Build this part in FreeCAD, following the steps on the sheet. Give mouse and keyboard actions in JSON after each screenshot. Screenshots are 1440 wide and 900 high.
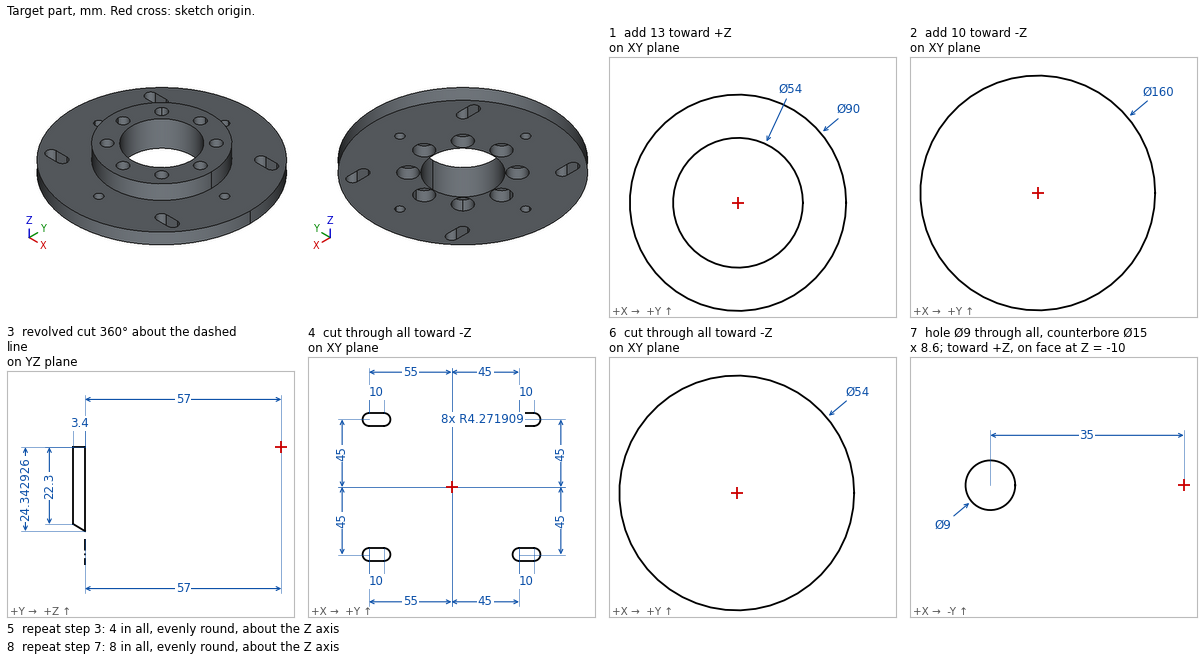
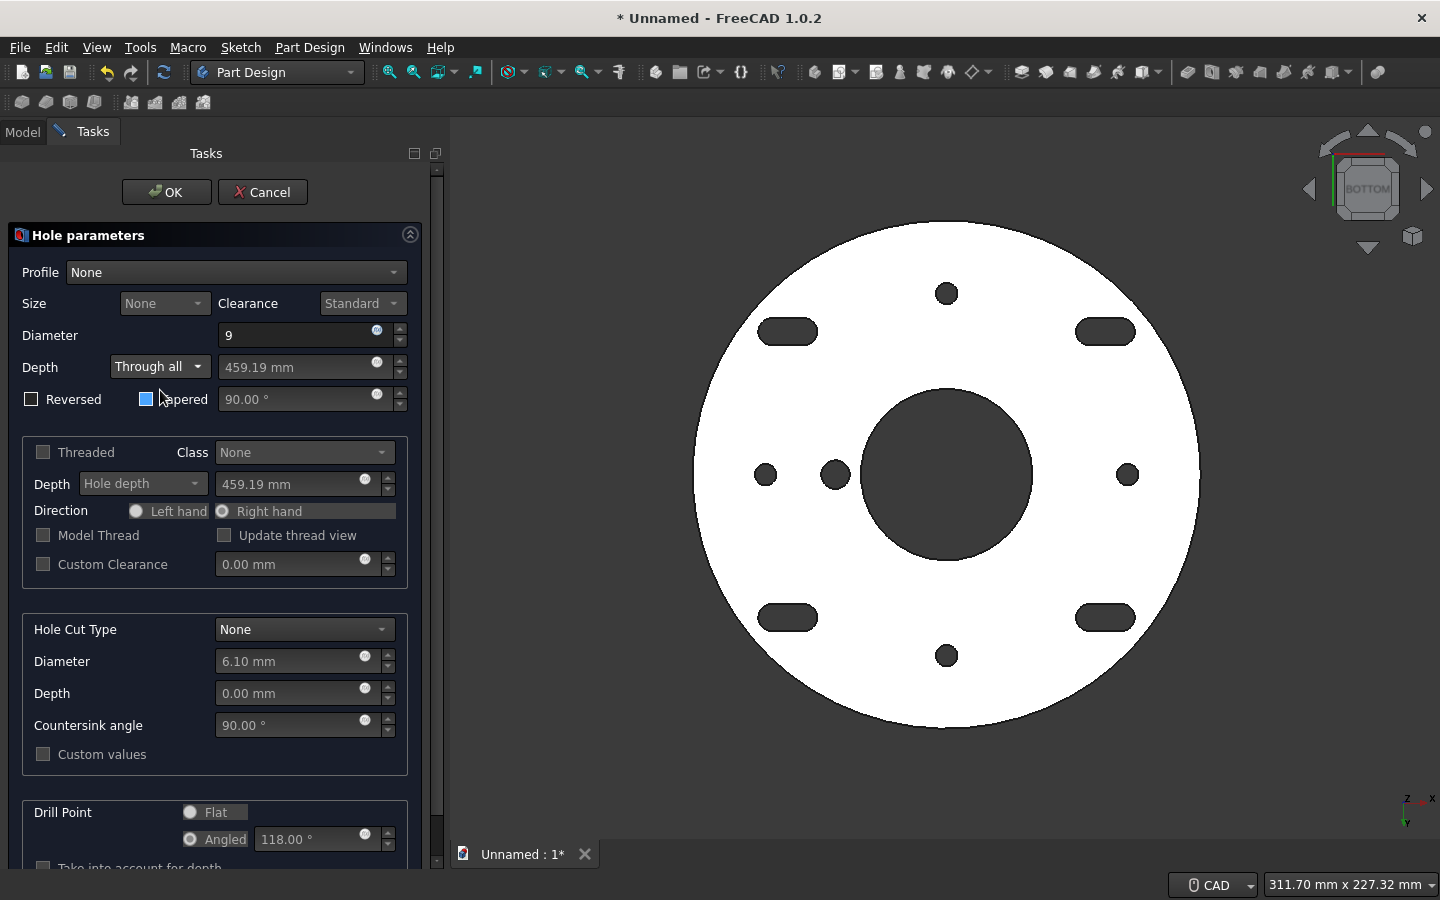
{"action": "left_click", "coordinate": [306, 630]}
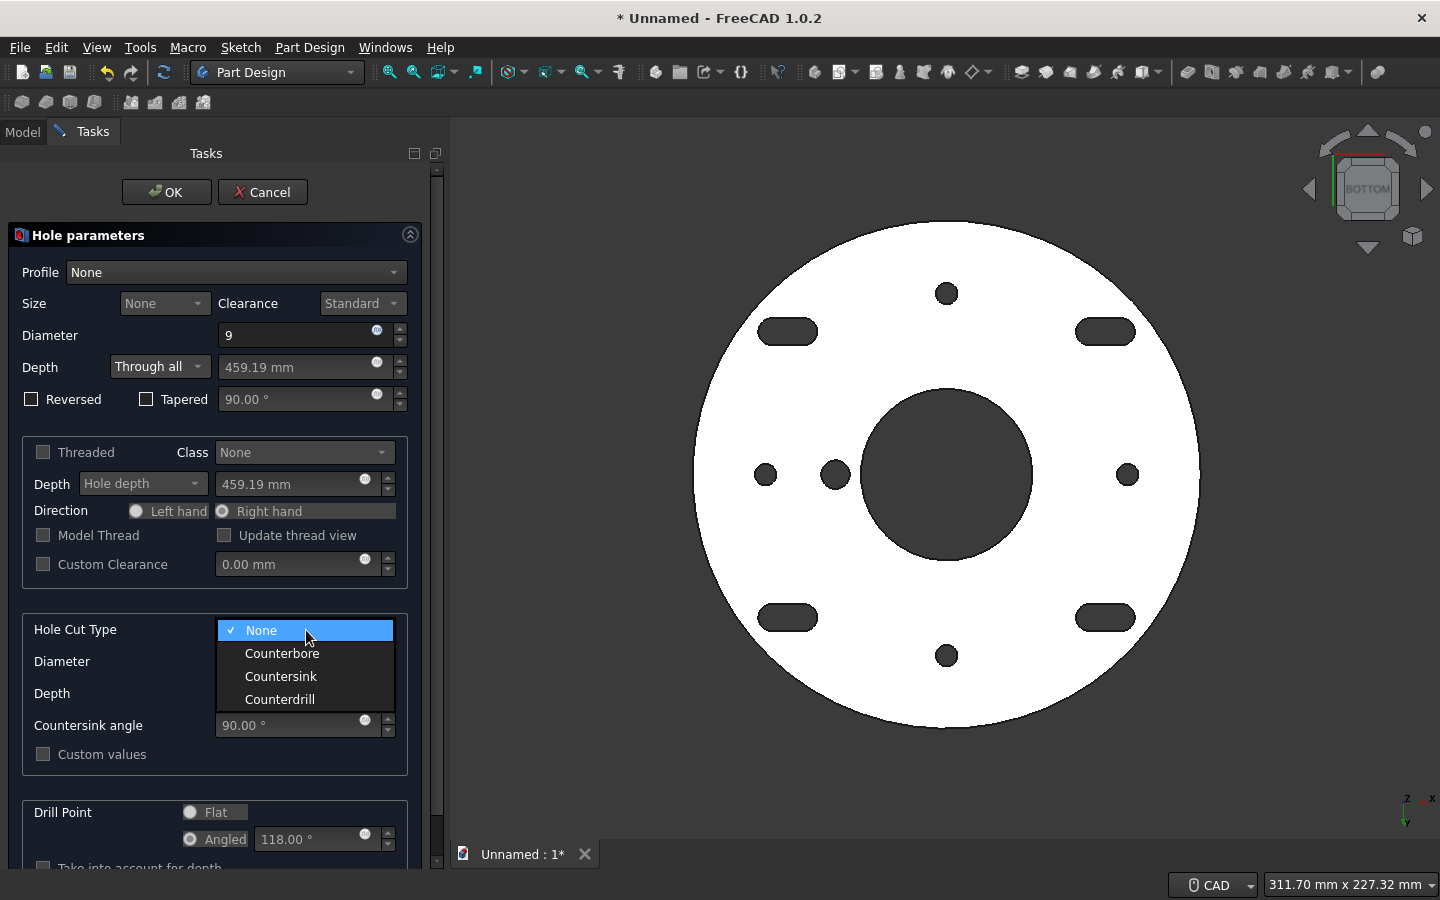
{"action": "left_click", "coordinate": [304, 654]}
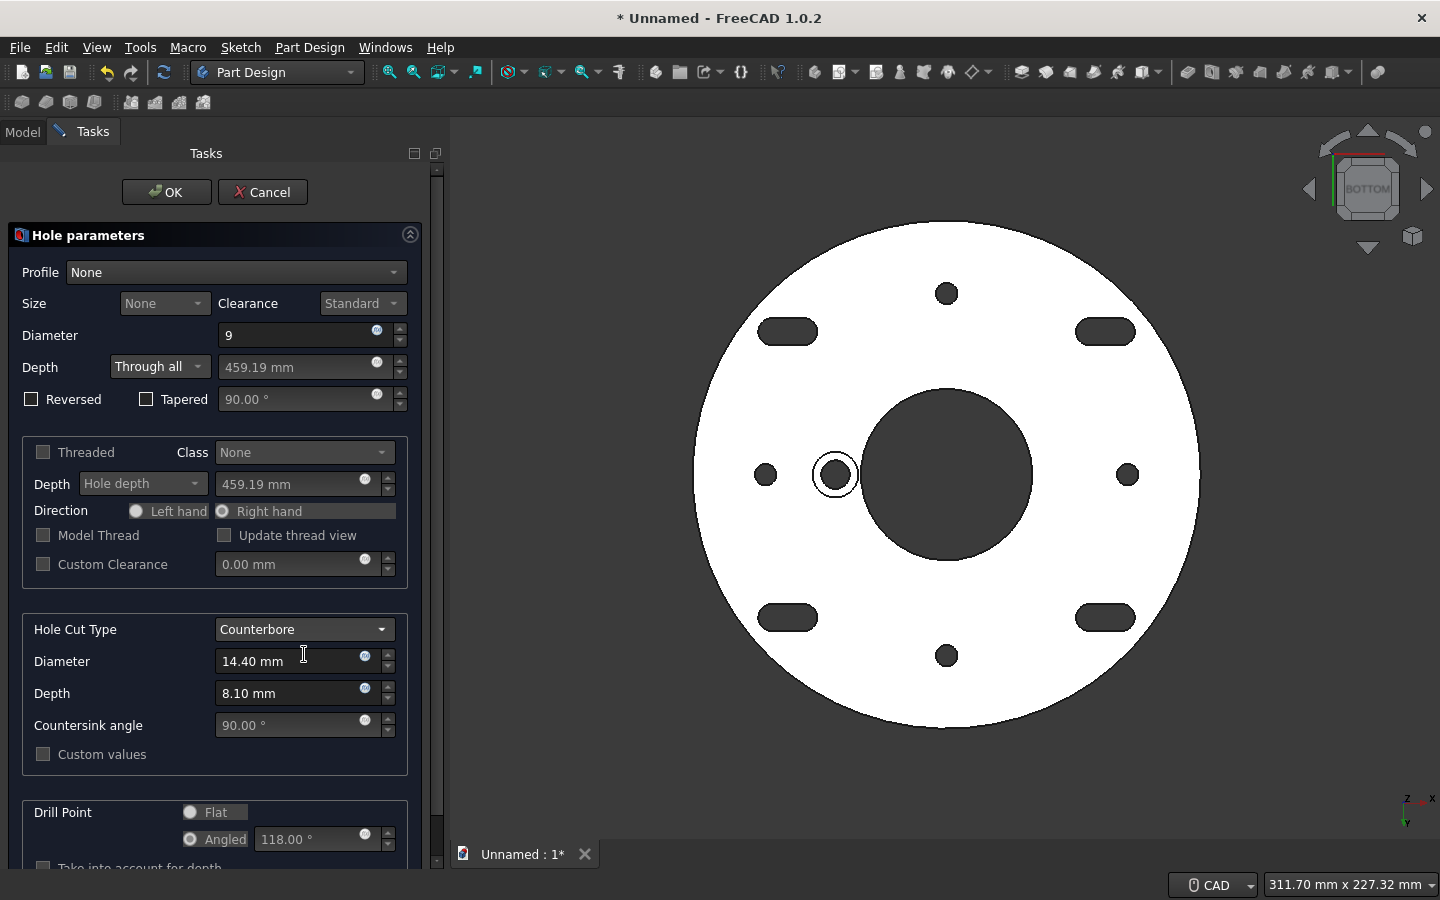
{"action": "triple_click", "coordinate": [298, 661]}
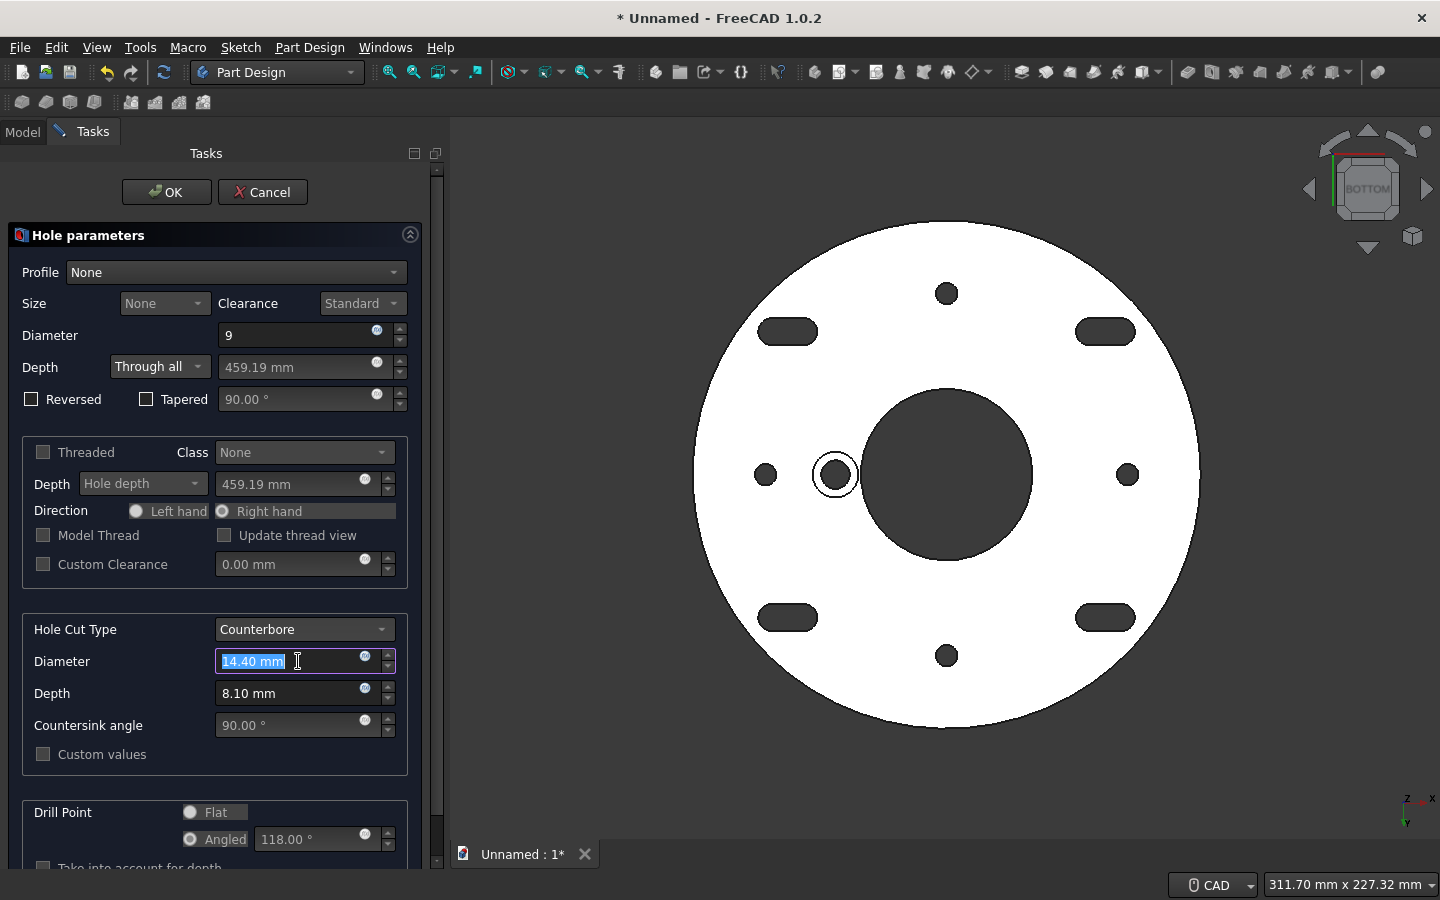
{"action": "type", "text": "15"}
{"action": "key", "text": "Tab"}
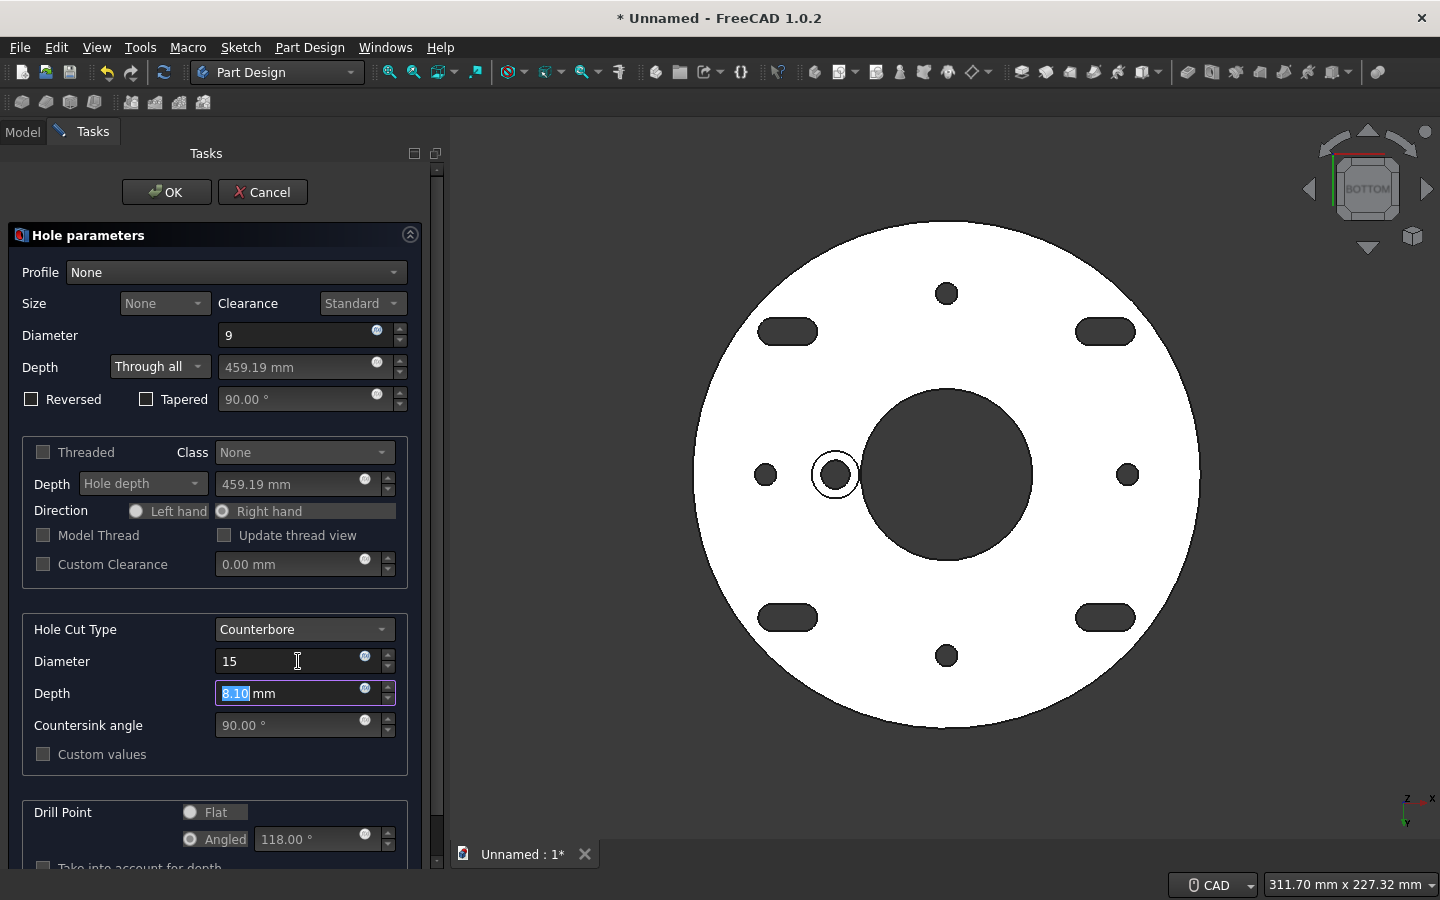
{"action": "type", "text": "8.6"}
{"action": "key", "text": "Tab"}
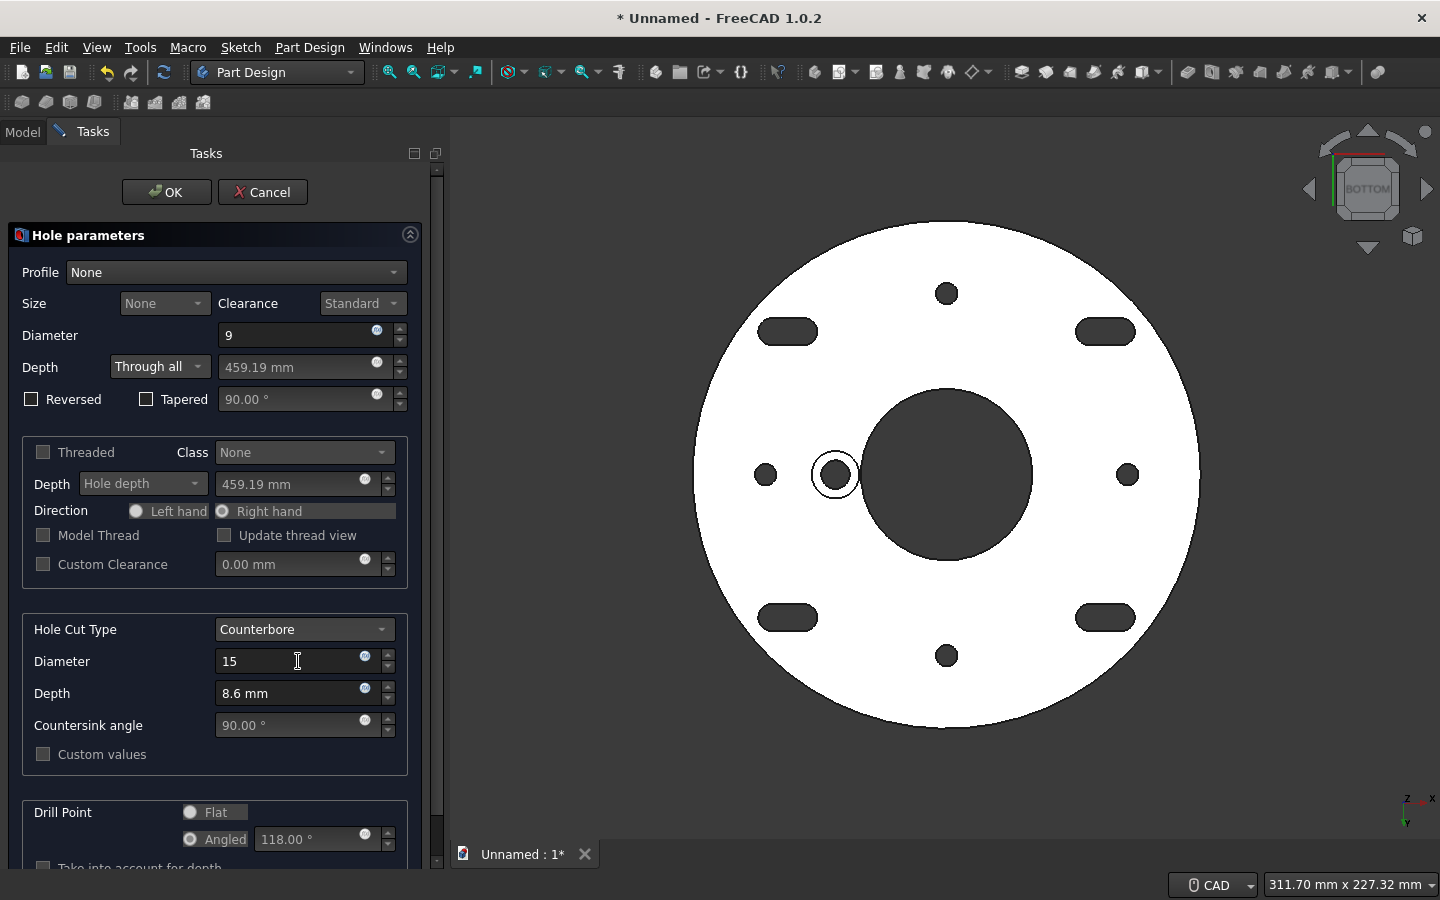
{"action": "left_click", "coordinate": [167, 192]}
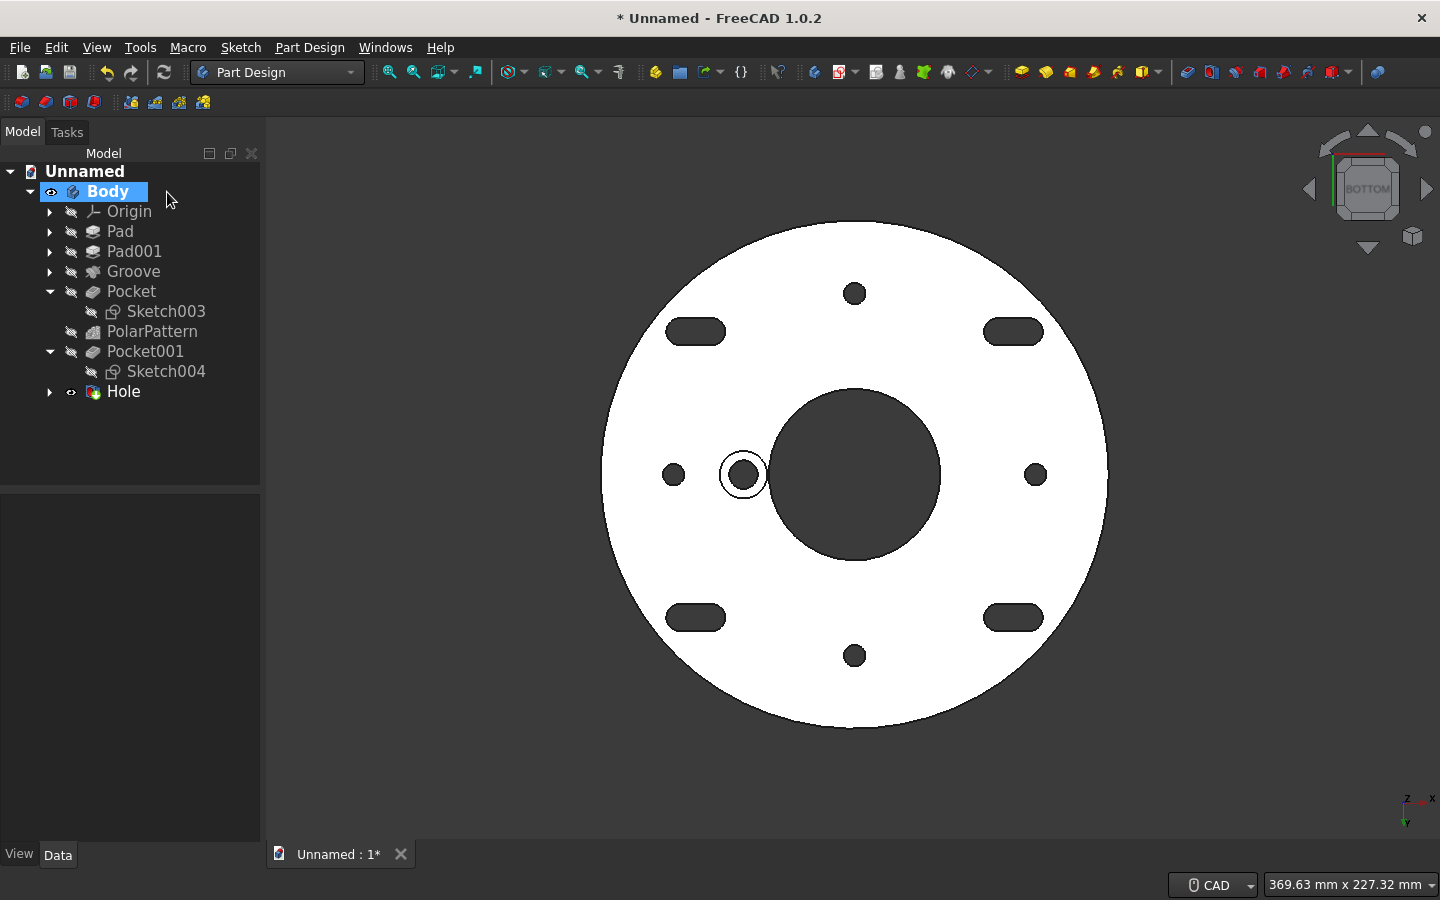
{"action": "left_click", "coordinate": [116, 392]}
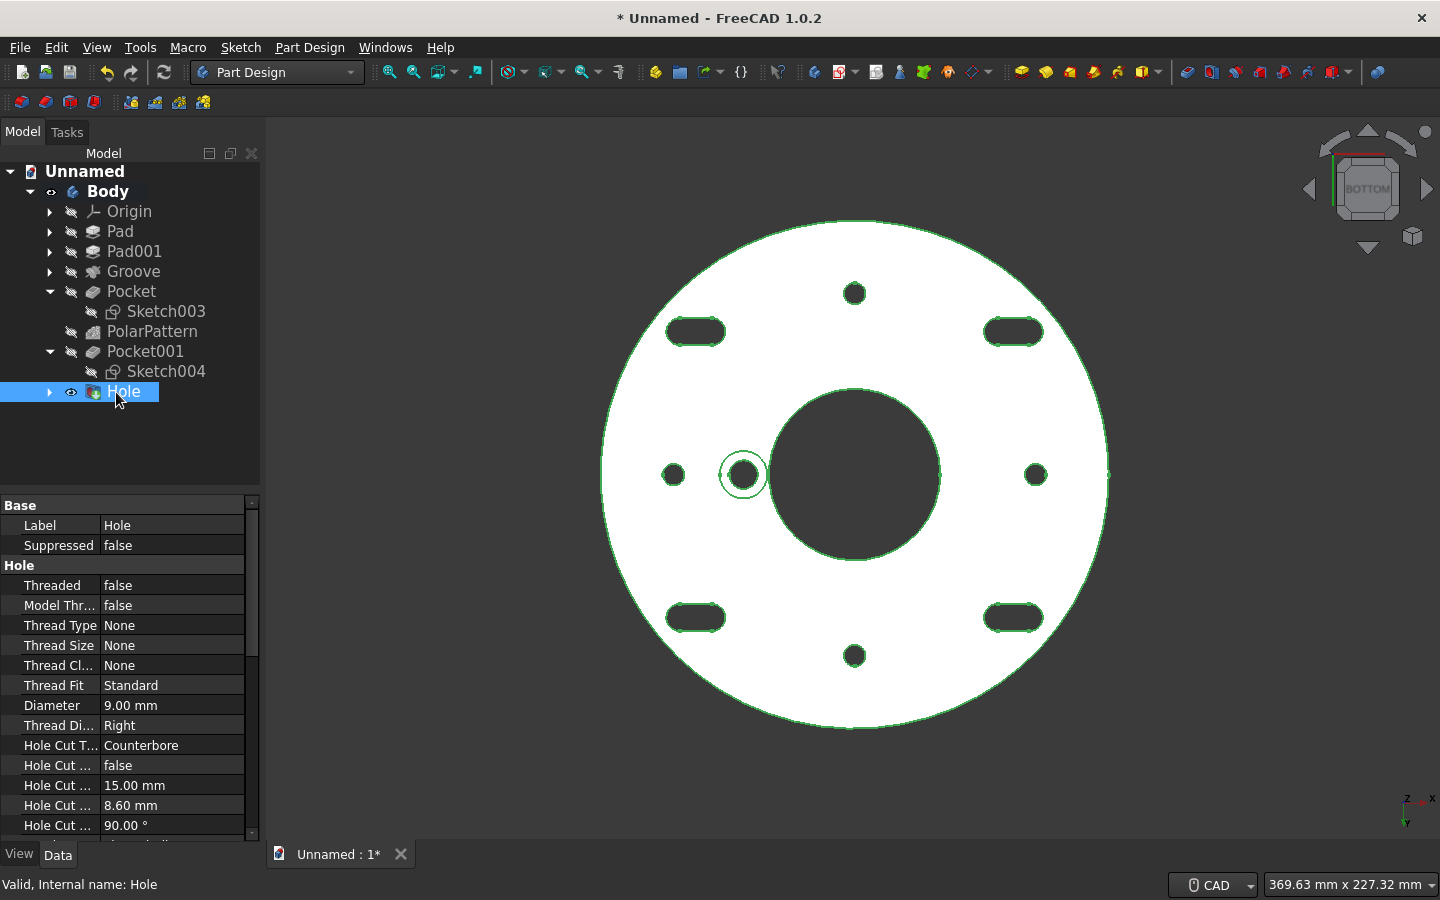
{"action": "left_click", "coordinate": [180, 102]}